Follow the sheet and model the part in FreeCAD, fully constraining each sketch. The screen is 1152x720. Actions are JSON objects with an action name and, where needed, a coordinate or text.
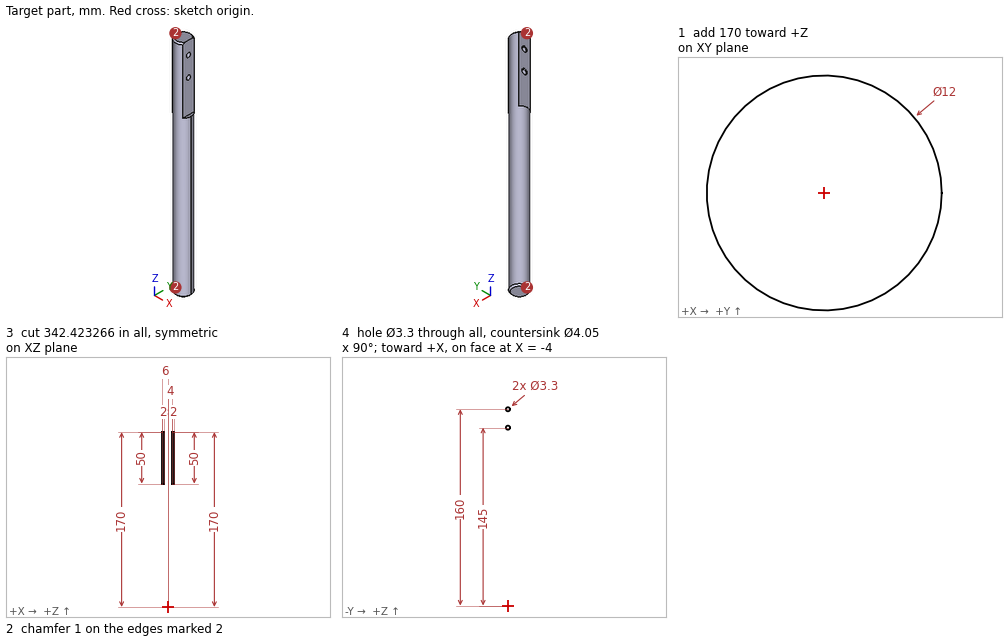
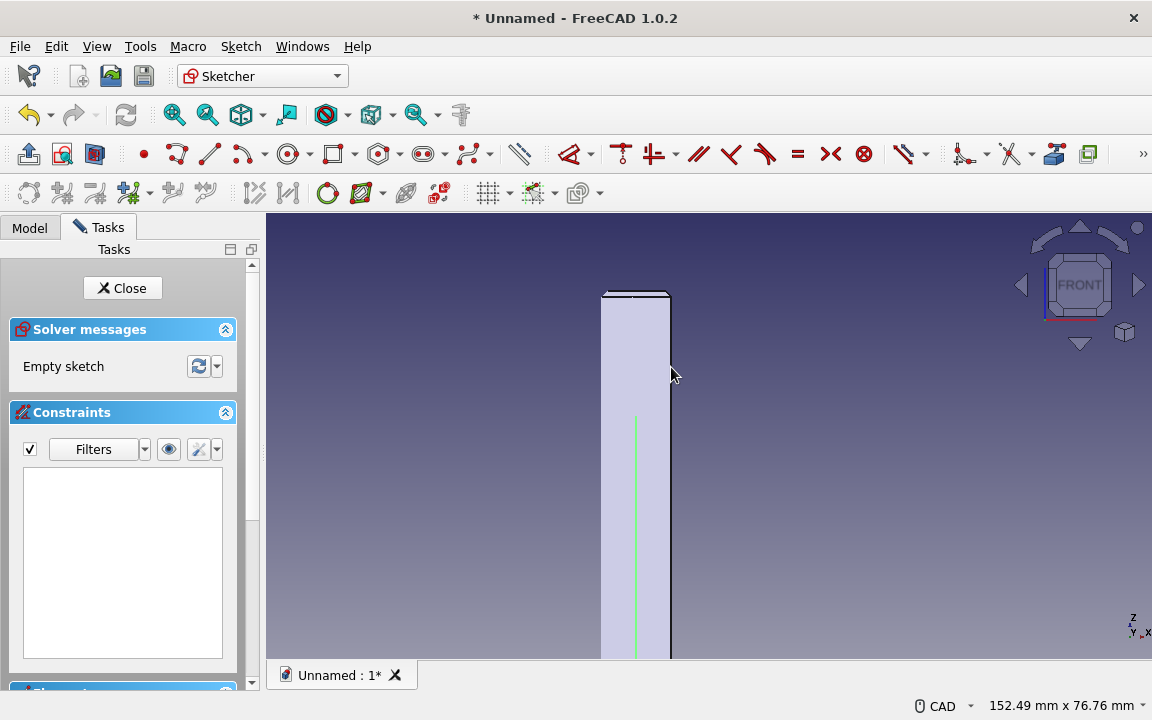
{"action": "key", "text": "g r"}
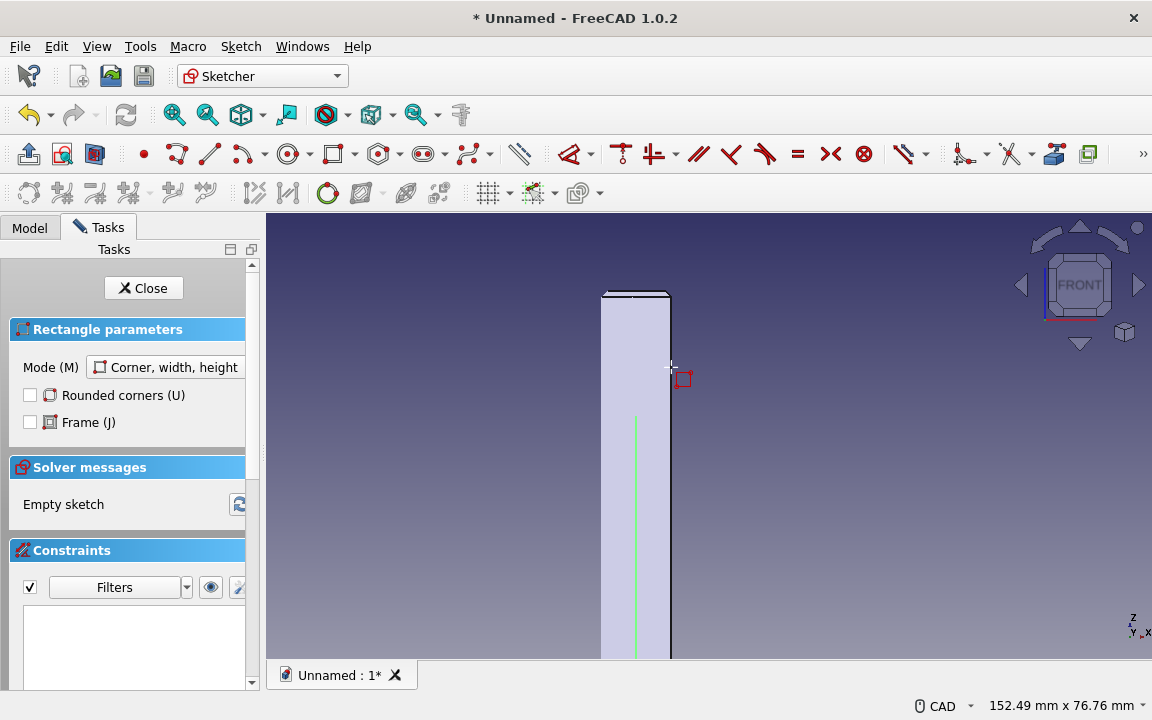
{"action": "scroll", "coordinate": [601, 291], "scroll_direction": "up", "scroll_amount": 2}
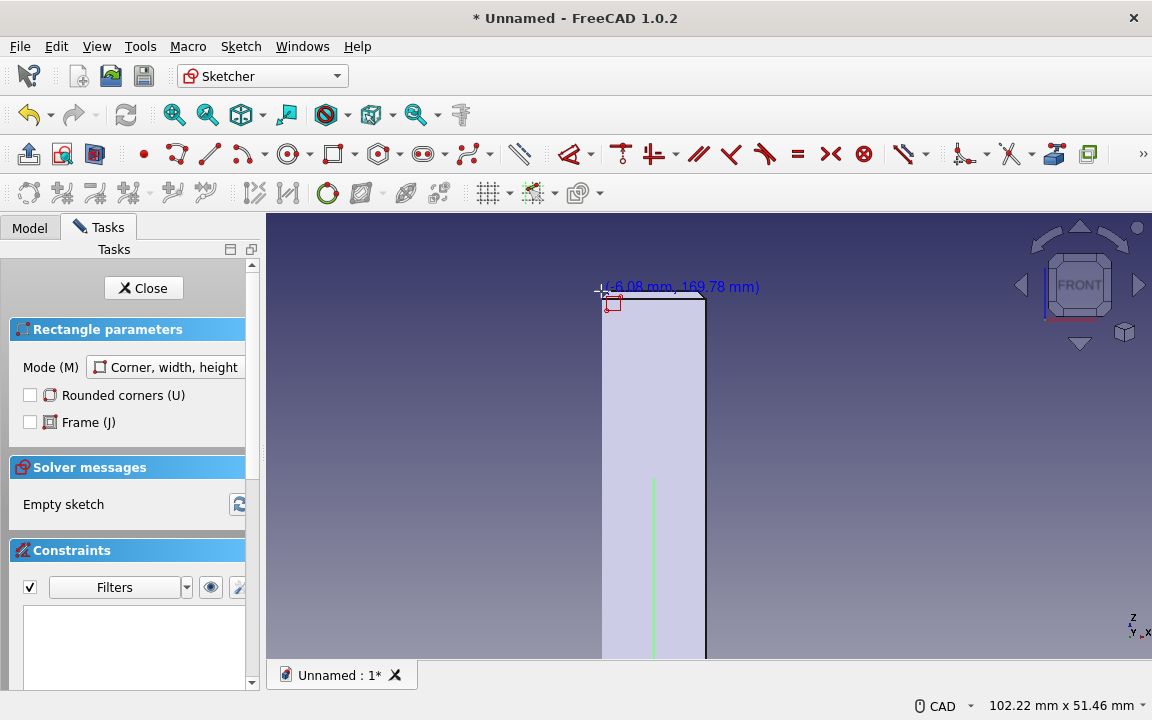
{"action": "left_click", "coordinate": [602, 291]}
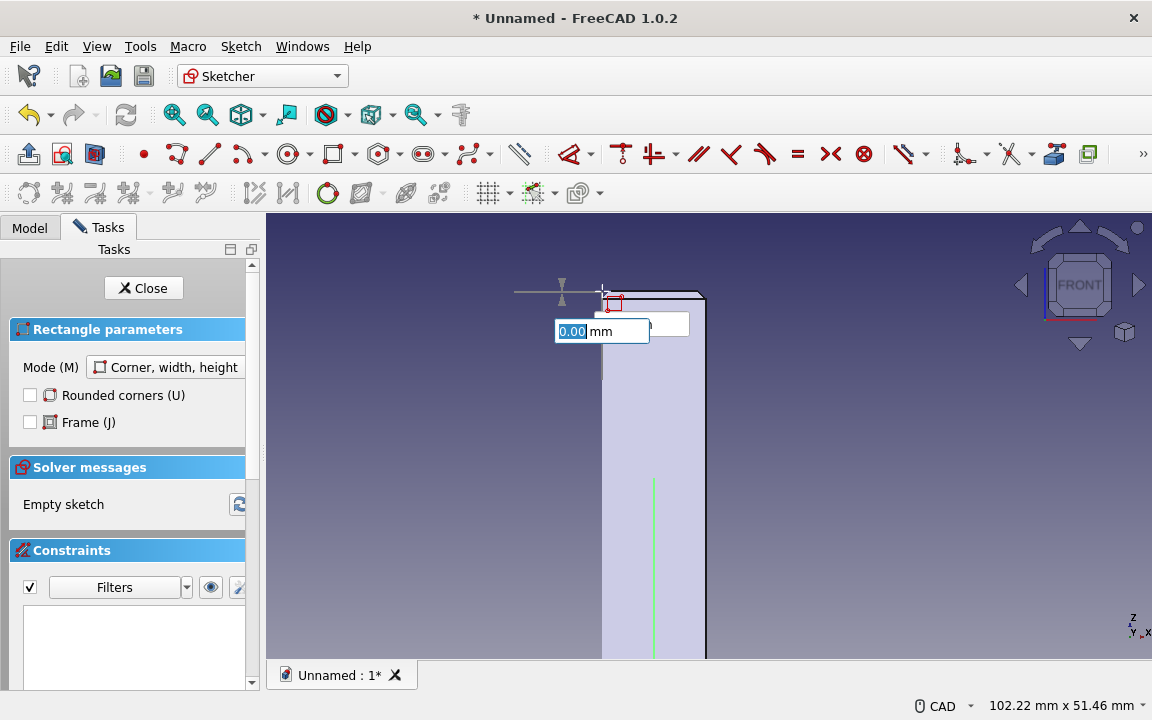
{"action": "scroll", "coordinate": [614, 291], "scroll_direction": "down", "scroll_amount": 2}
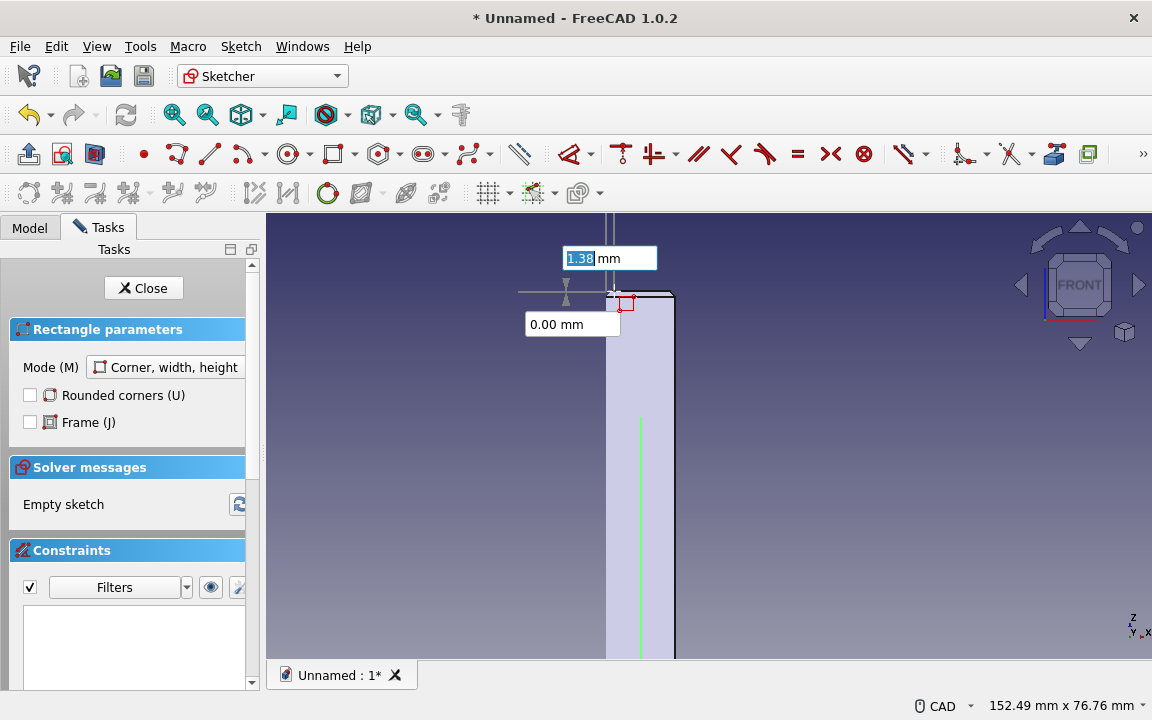
{"action": "left_click", "coordinate": [617, 581]}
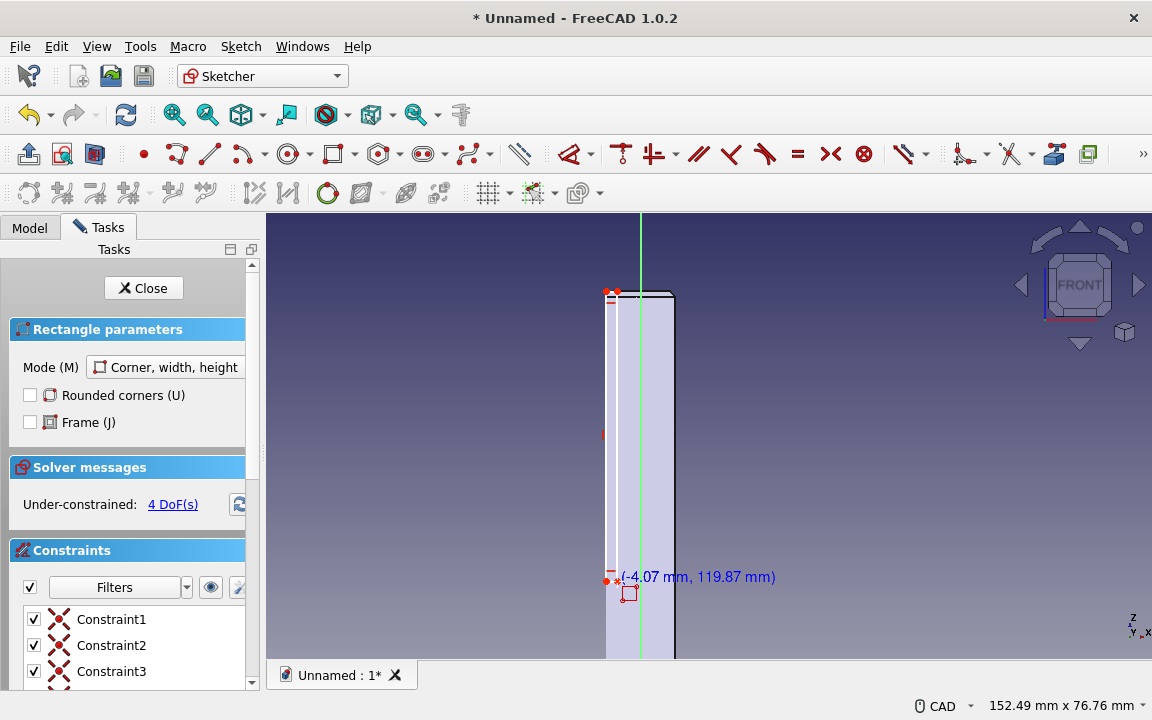
{"action": "scroll", "coordinate": [664, 291], "scroll_direction": "up", "scroll_amount": 2}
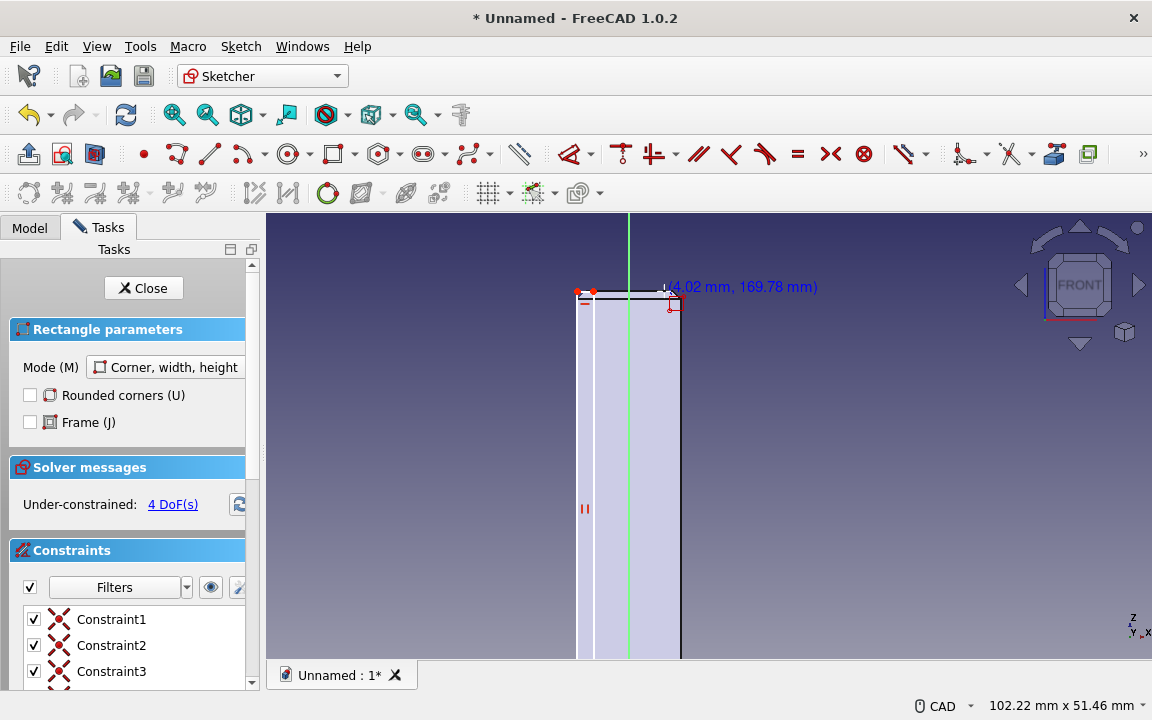
{"action": "left_click", "coordinate": [664, 291]}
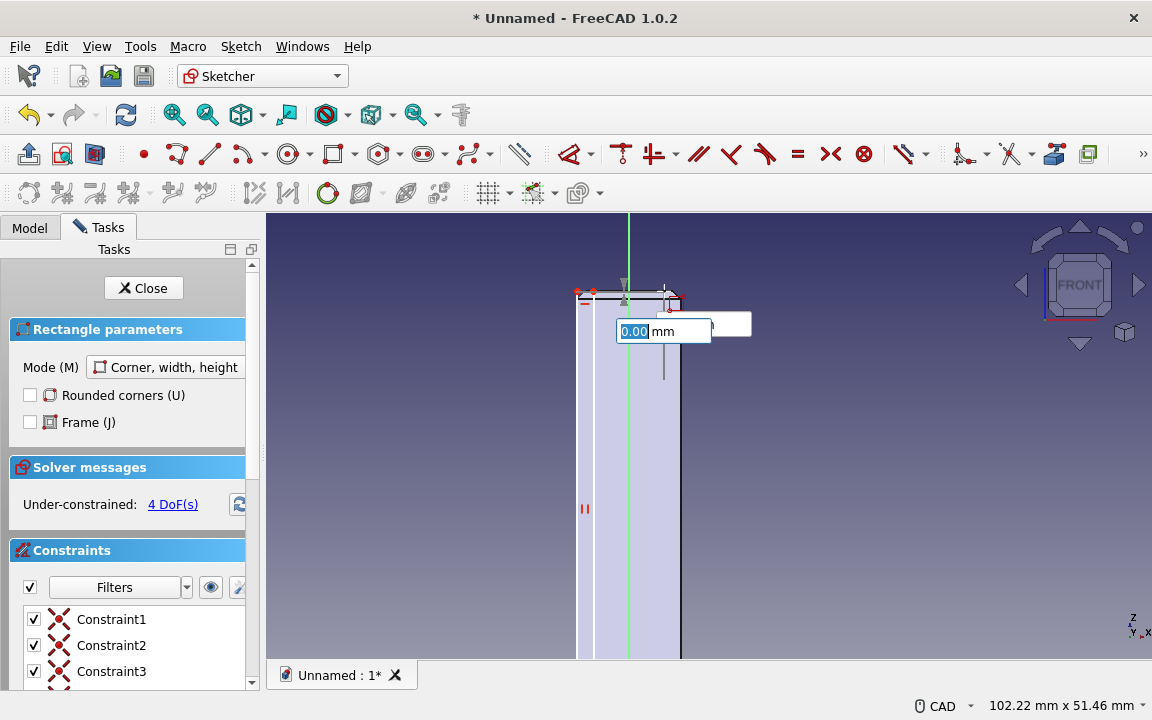
{"action": "scroll", "coordinate": [664, 291], "scroll_direction": "down", "scroll_amount": 2}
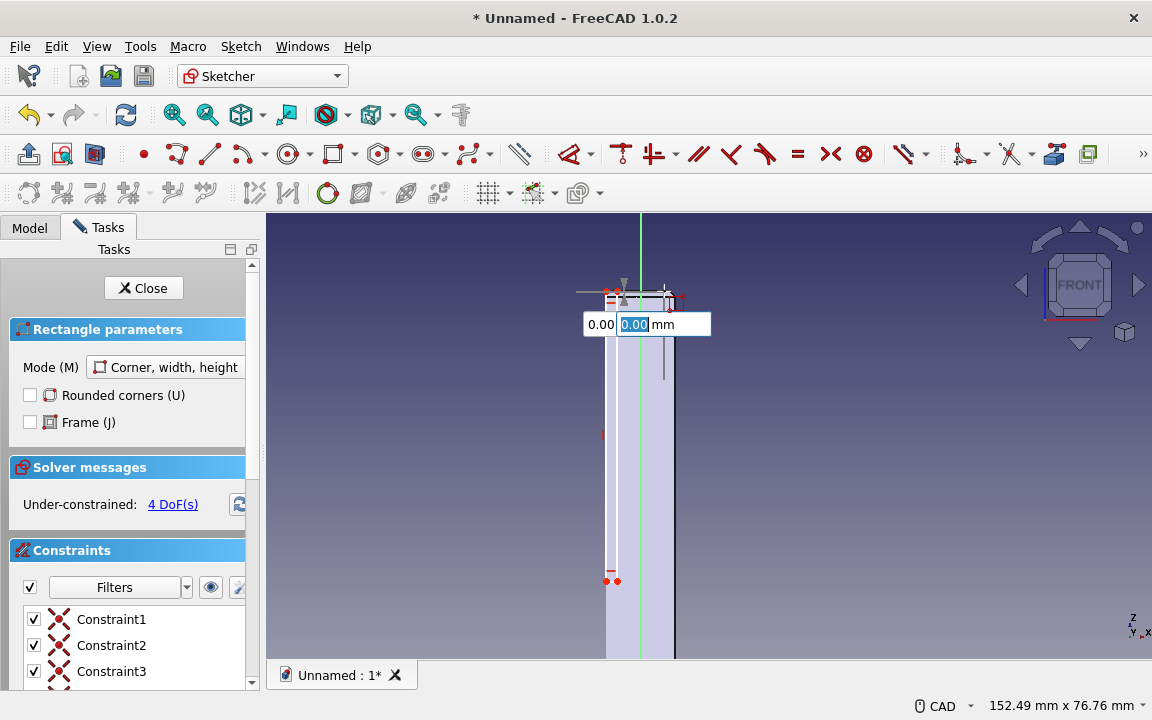
{"action": "left_click", "coordinate": [675, 581]}
{"action": "key", "text": "Escape"}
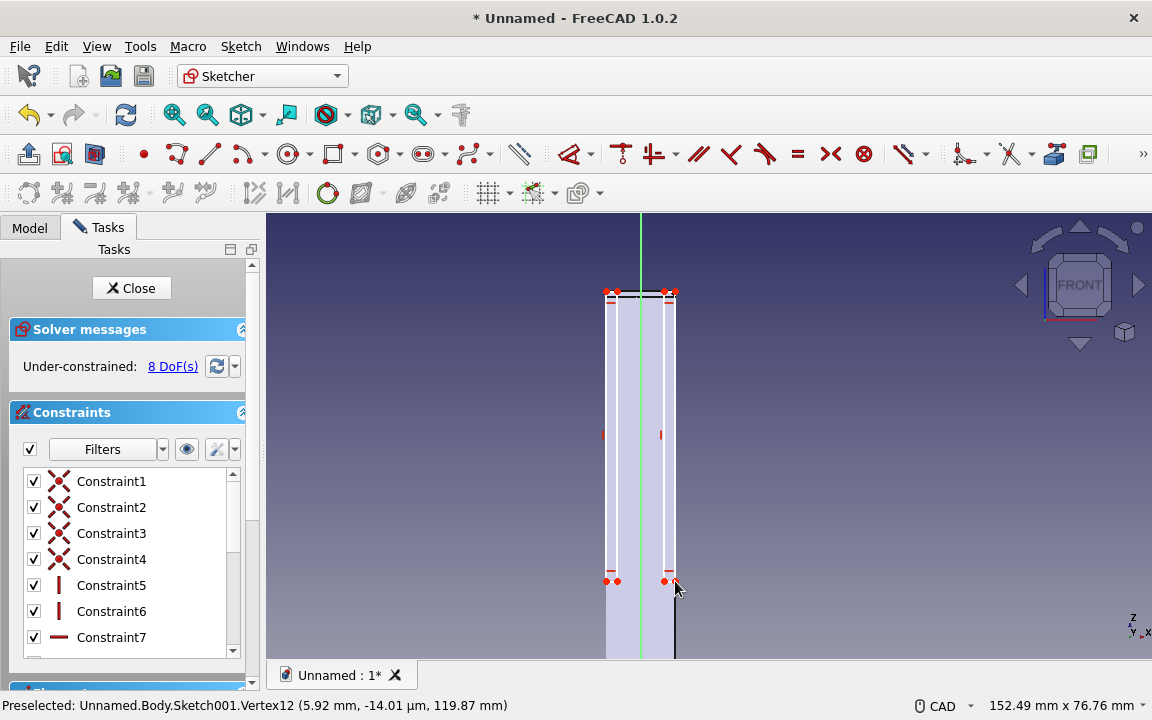
{"action": "key", "text": "d"}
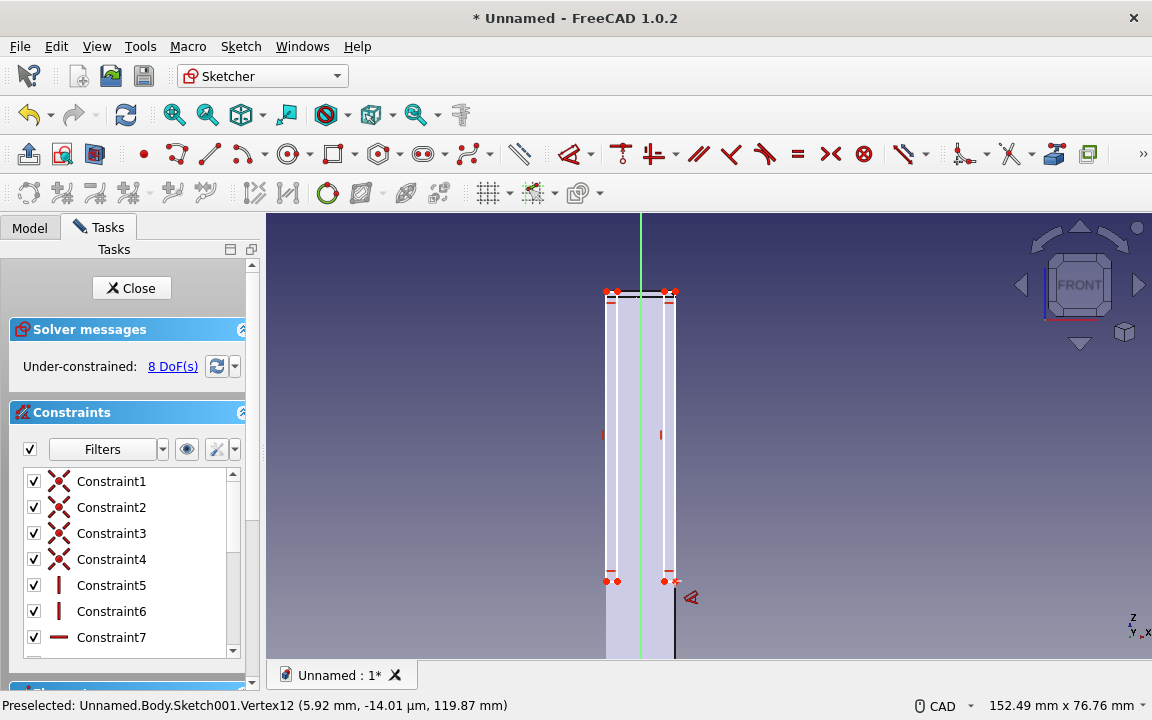
{"action": "scroll", "coordinate": [612, 582], "scroll_direction": "up", "scroll_amount": 7}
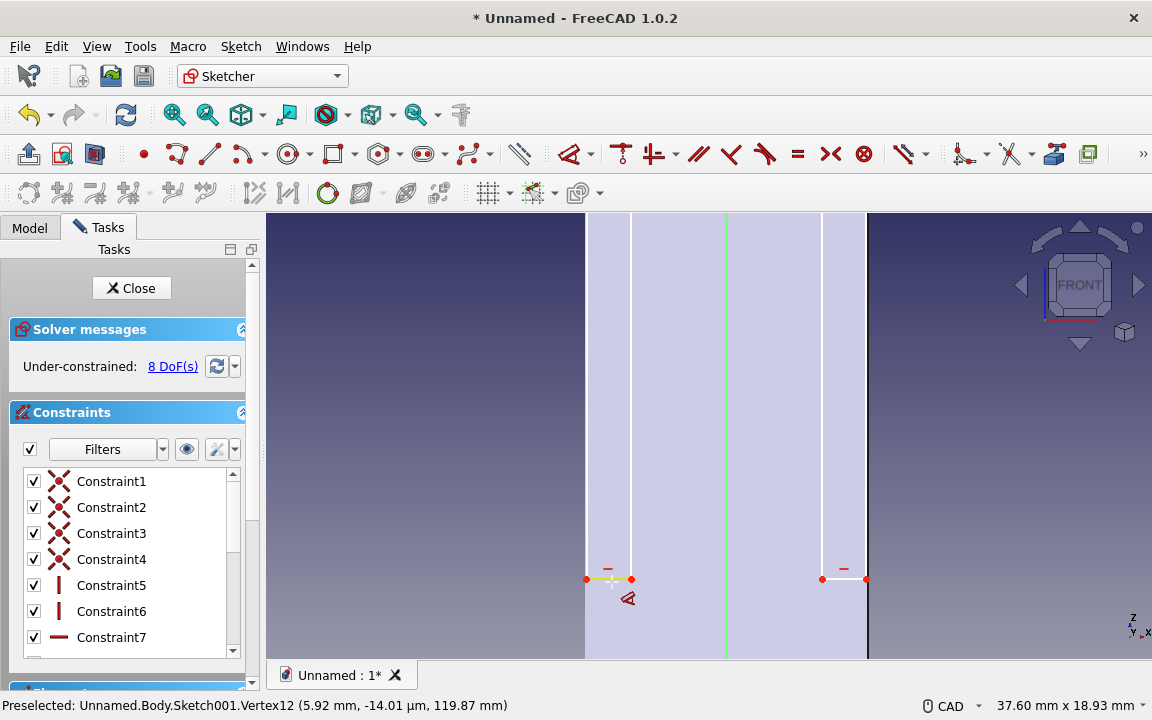
{"action": "left_click", "coordinate": [609, 579]}
{"action": "left_click", "coordinate": [609, 613]}